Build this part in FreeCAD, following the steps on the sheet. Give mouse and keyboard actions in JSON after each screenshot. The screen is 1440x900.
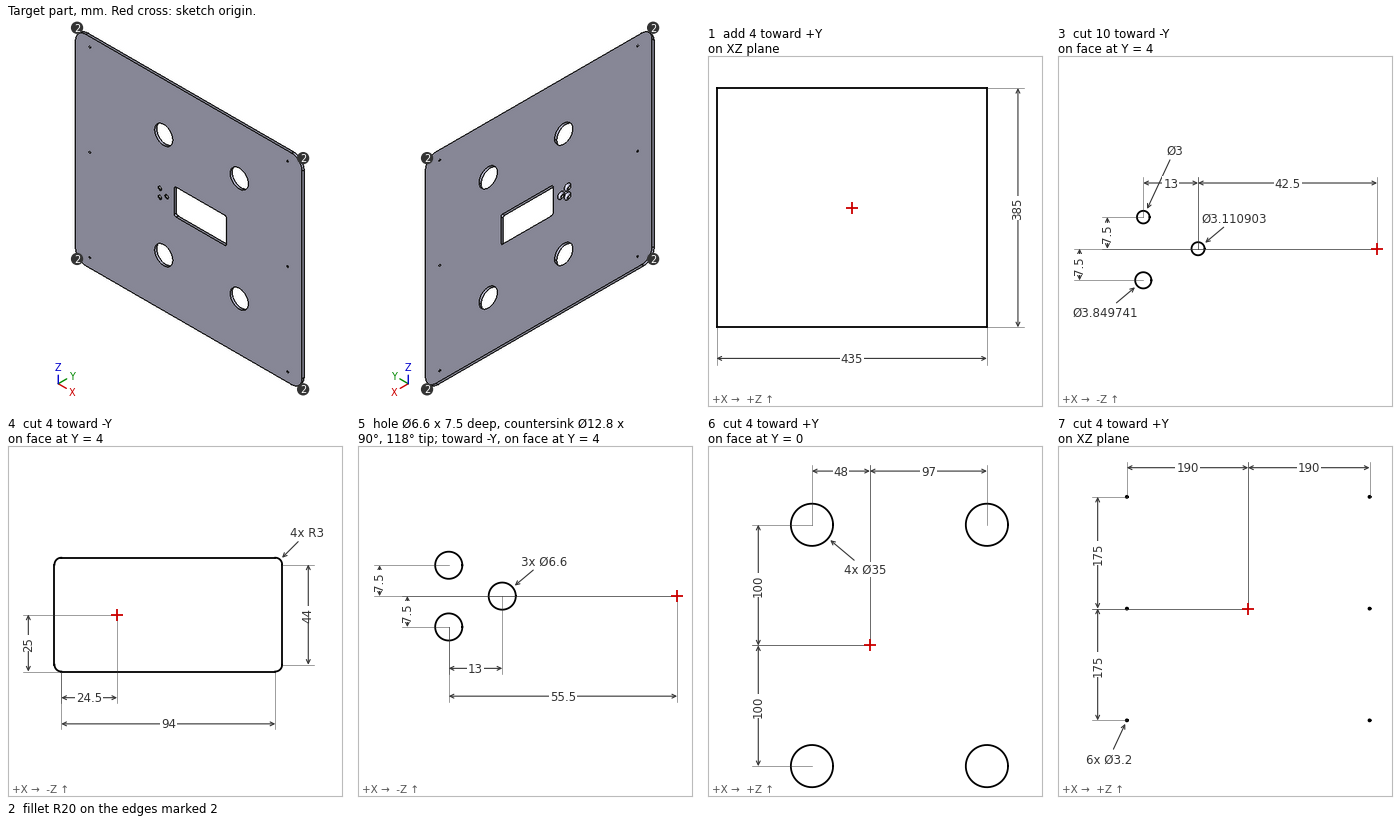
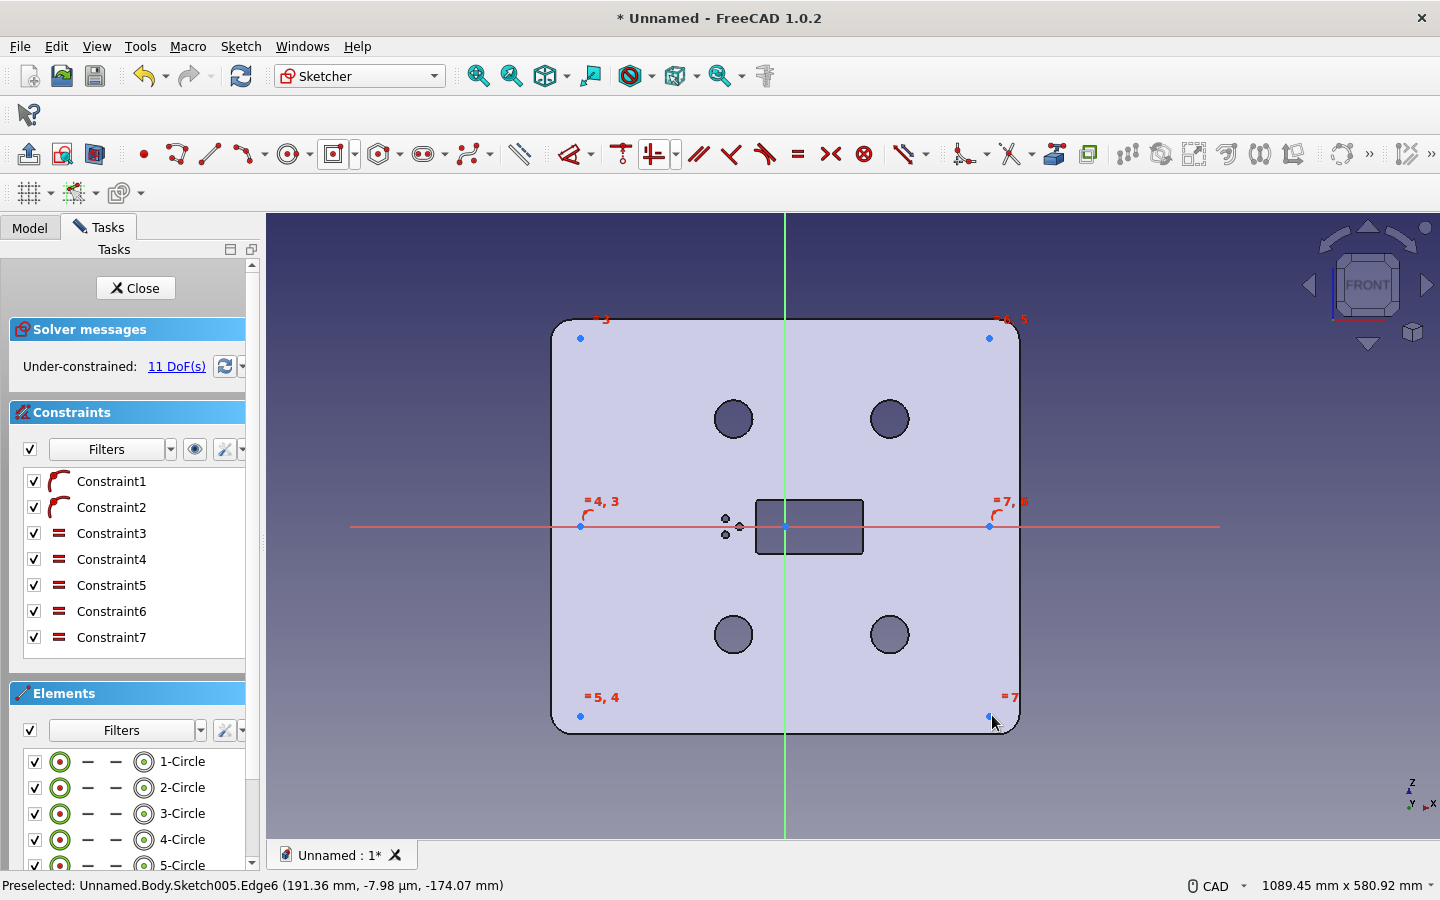
{"action": "left_click", "coordinate": [581, 339]}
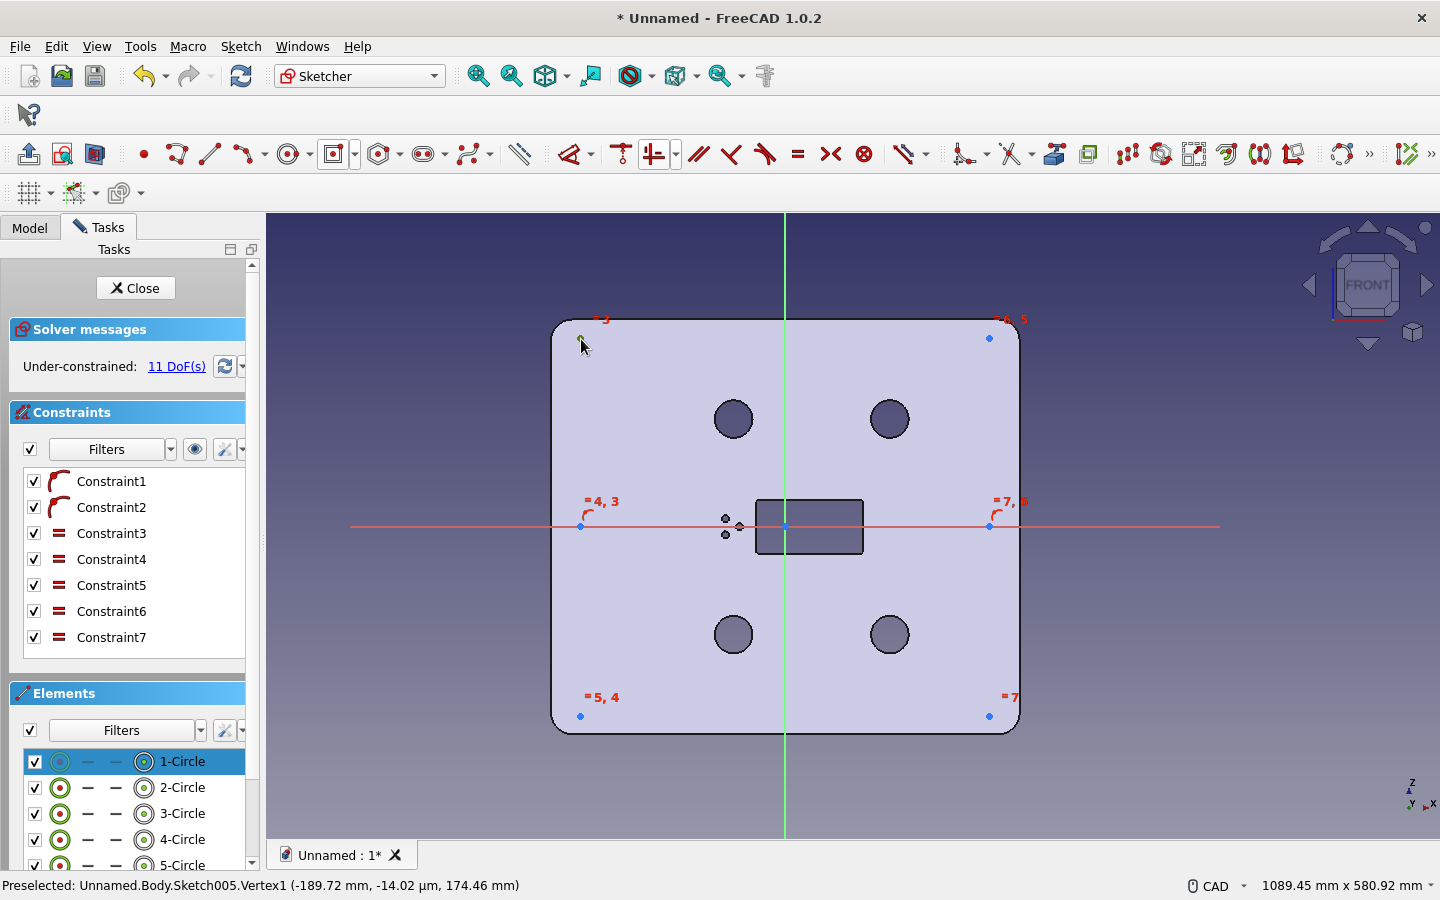
{"action": "left_click", "coordinate": [581, 527]}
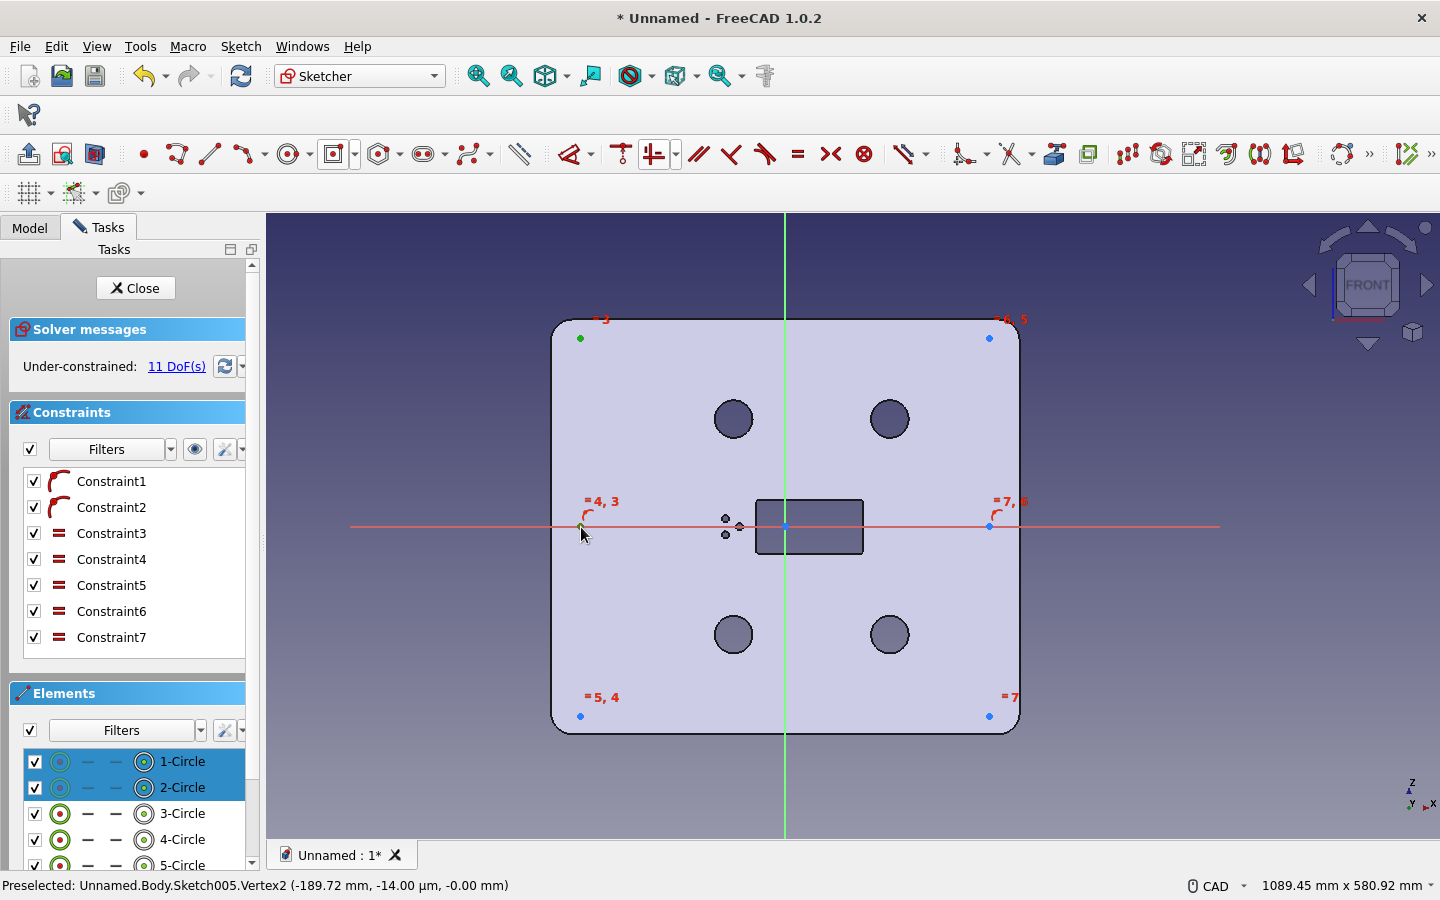
{"action": "left_click", "coordinate": [676, 154]}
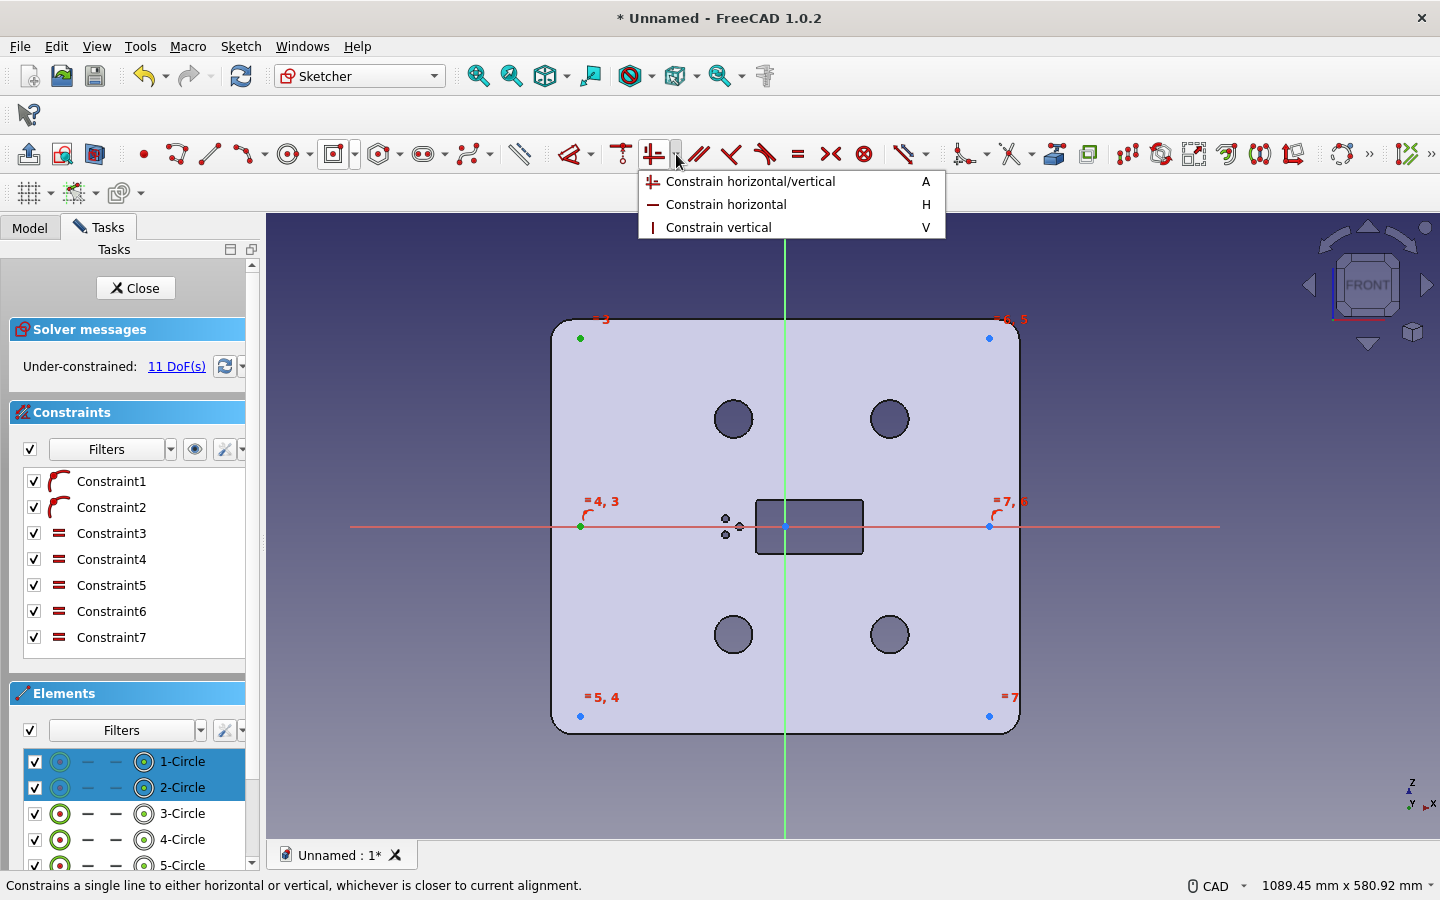
{"action": "left_click", "coordinate": [792, 228]}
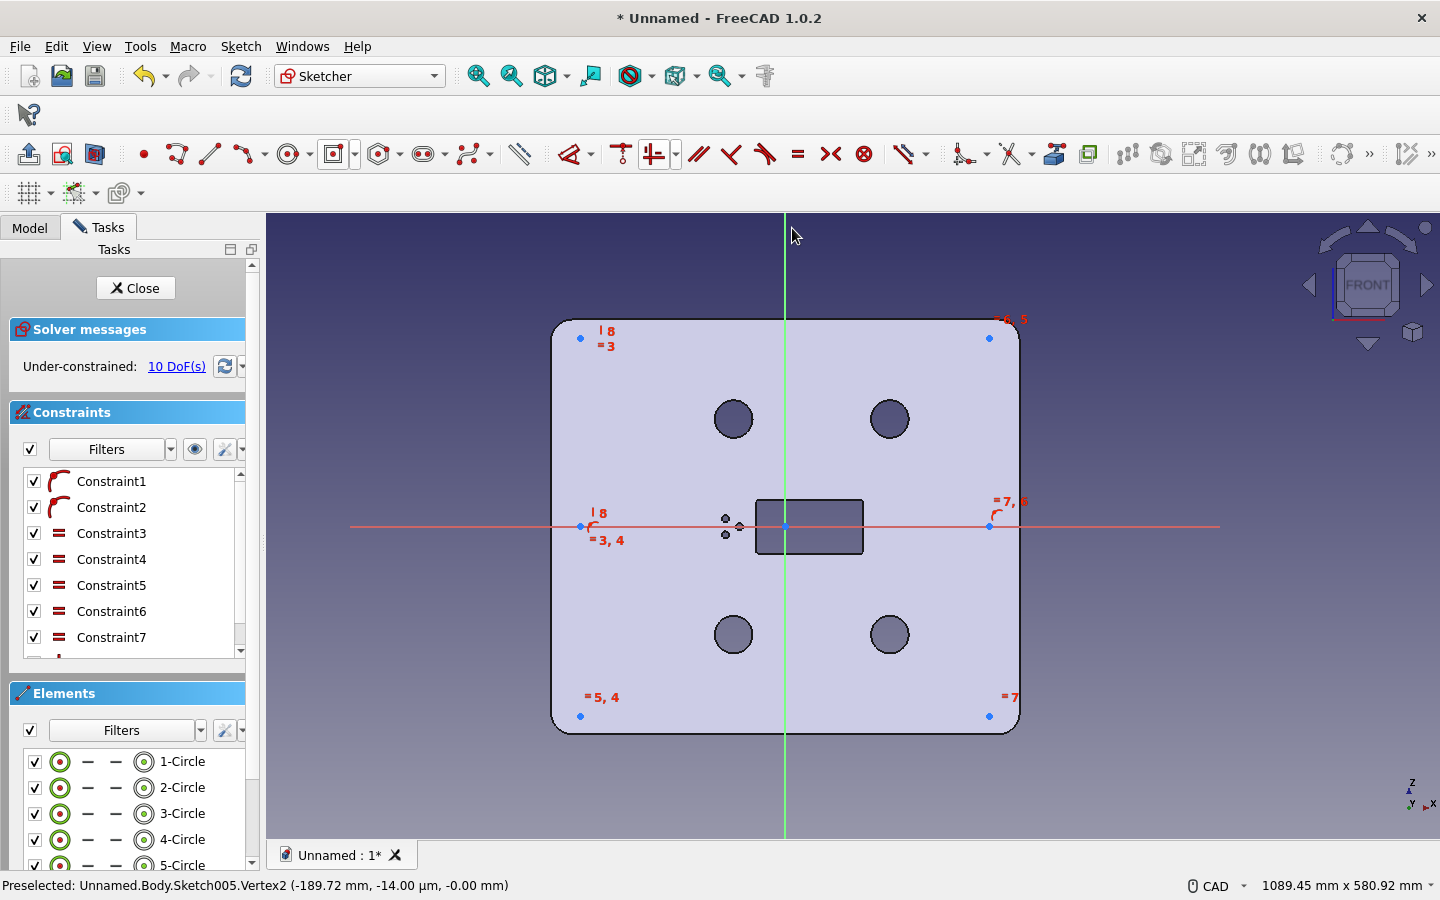
{"action": "left_click", "coordinate": [581, 527]}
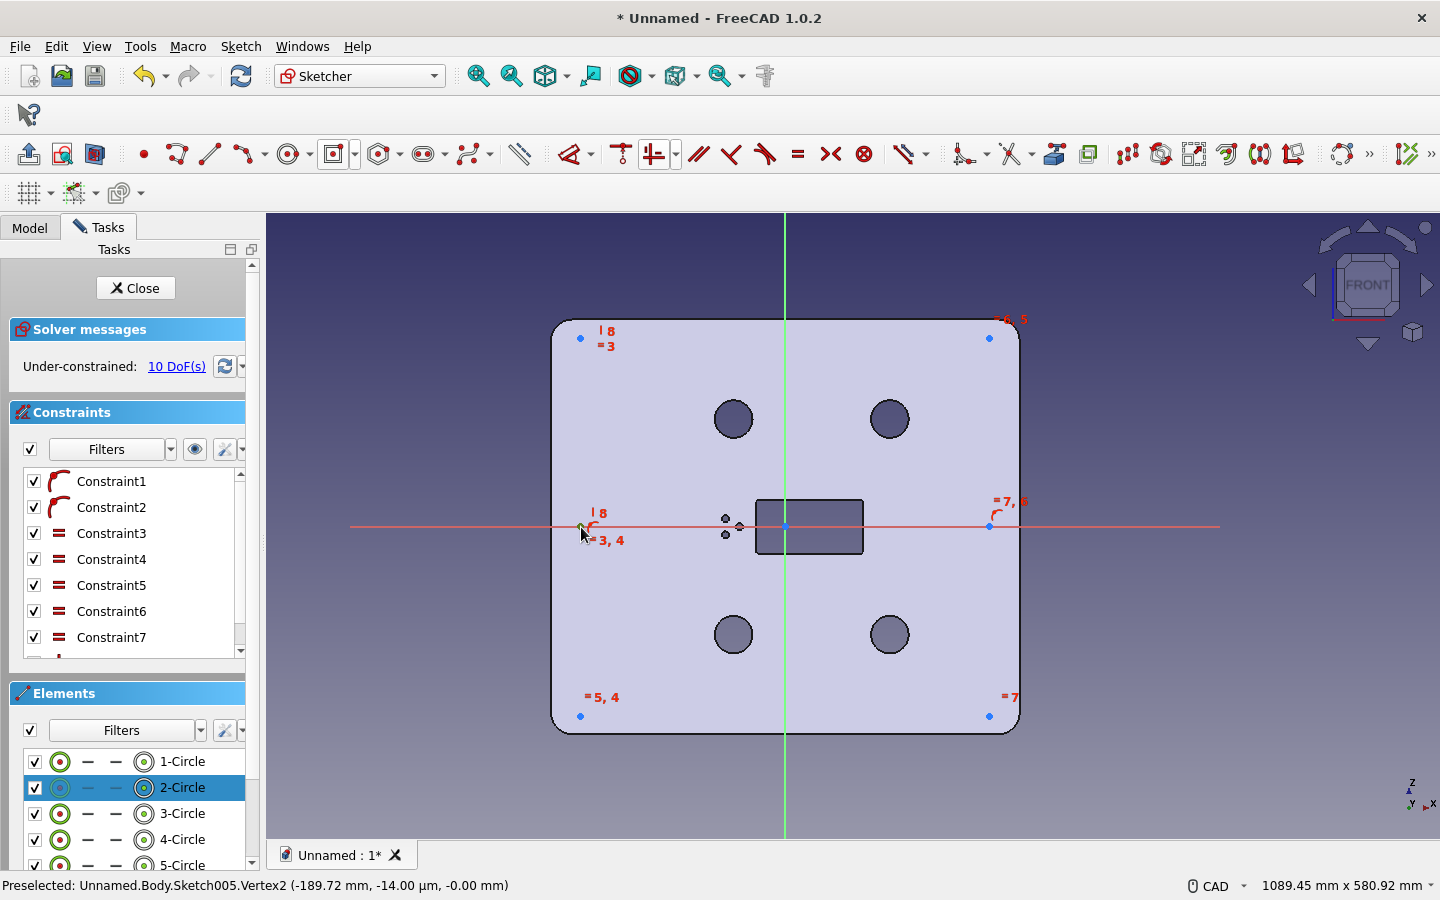
{"action": "left_click", "coordinate": [581, 717]}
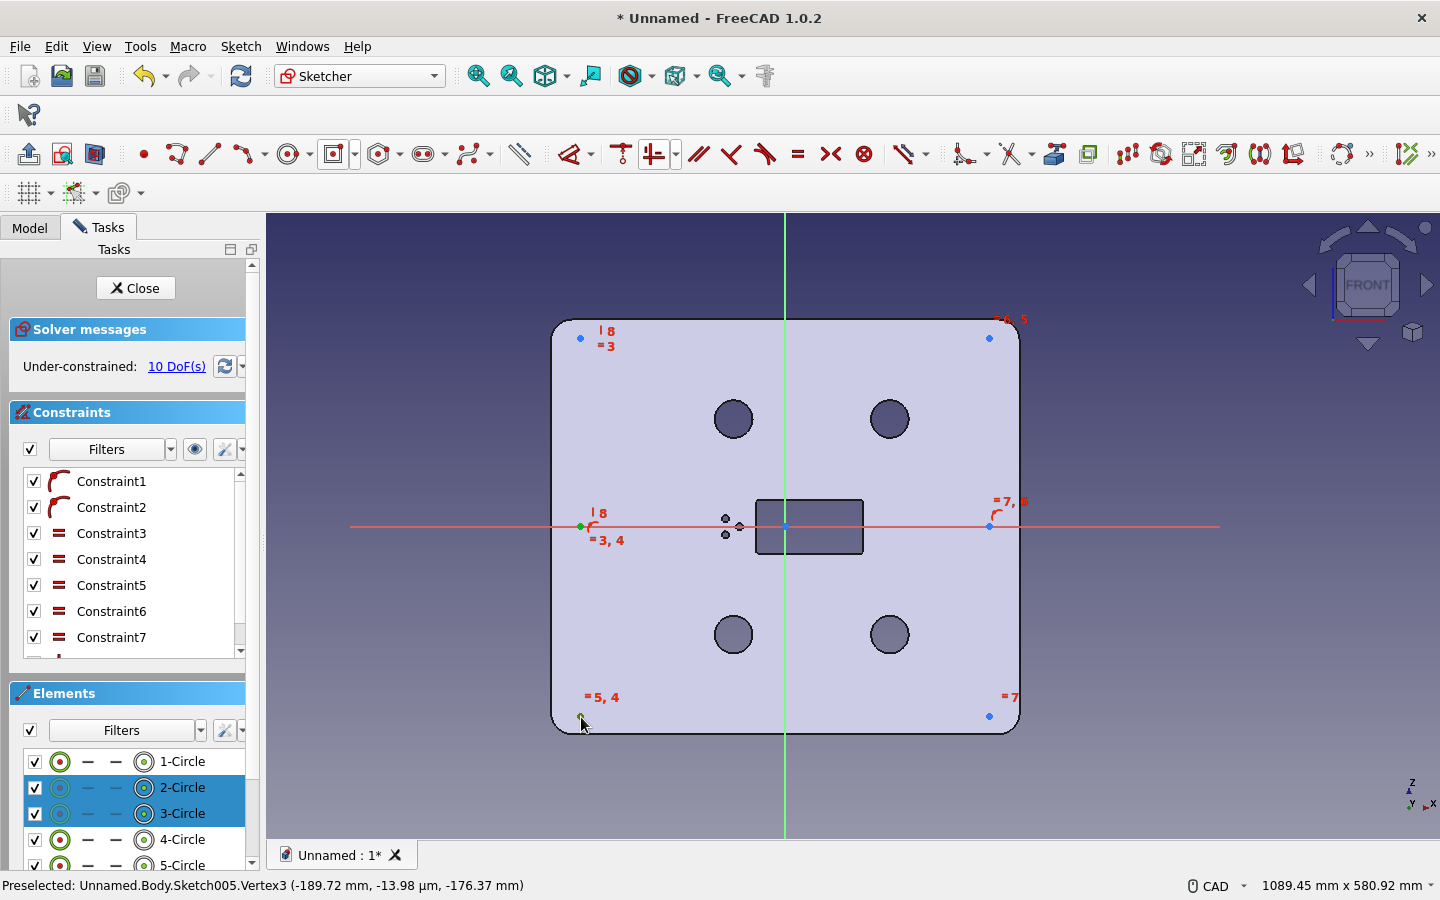
{"action": "left_click", "coordinate": [676, 154]}